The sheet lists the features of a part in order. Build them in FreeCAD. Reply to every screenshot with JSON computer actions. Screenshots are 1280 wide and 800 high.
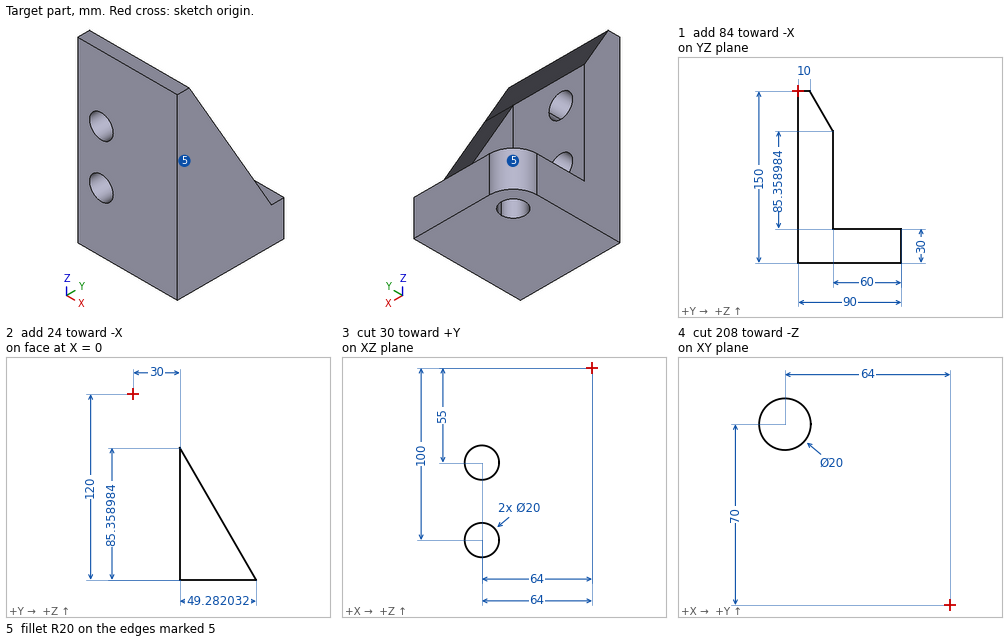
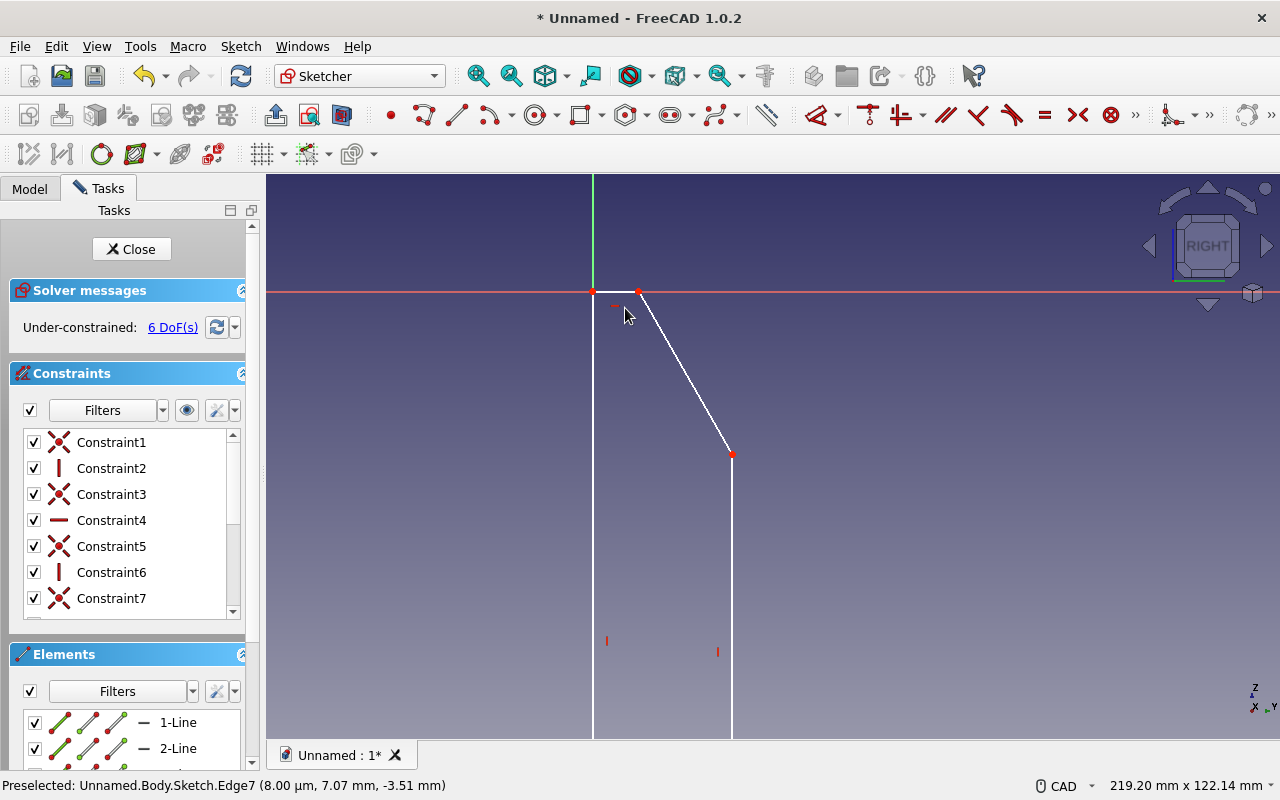
{"action": "left_click", "coordinate": [816, 116]}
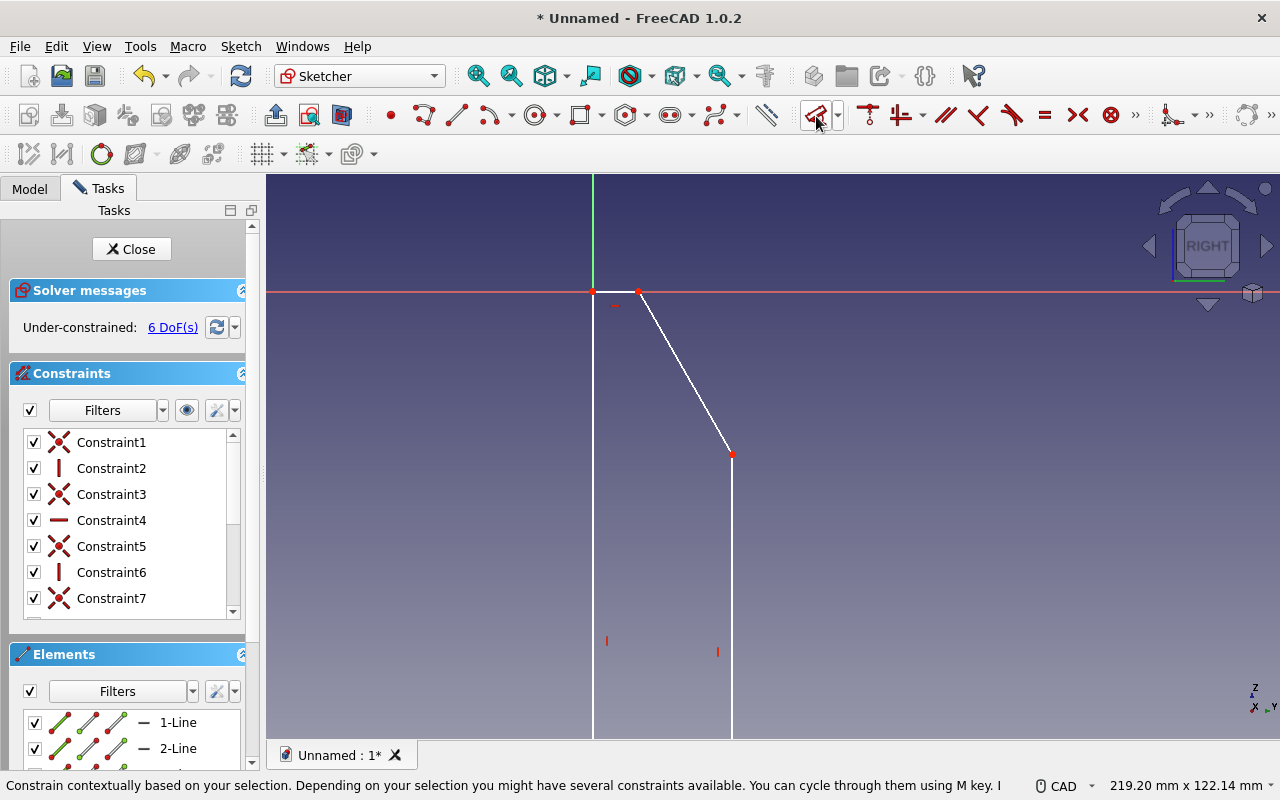
{"action": "scroll", "coordinate": [587, 235], "scroll_direction": "down", "scroll_amount": 3}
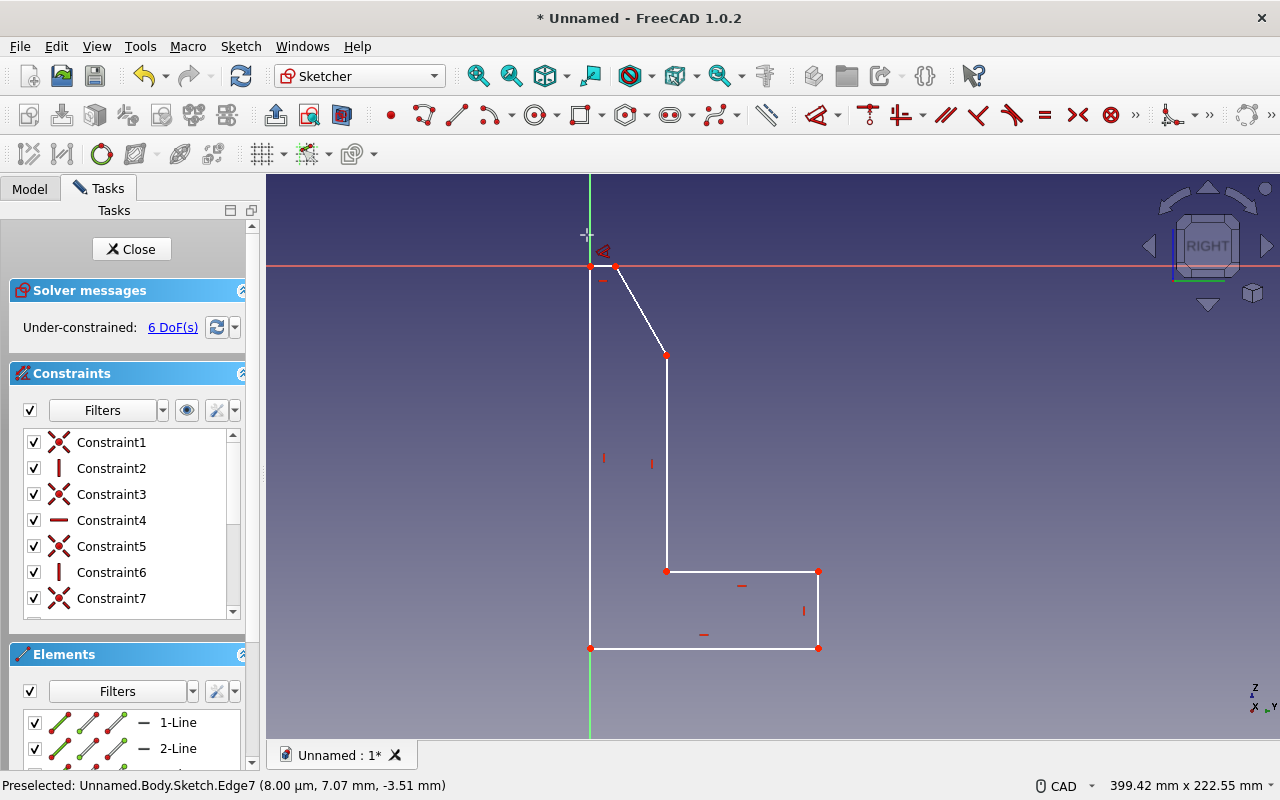
{"action": "left_click", "coordinate": [659, 649]}
{"action": "left_click", "coordinate": [704, 683]}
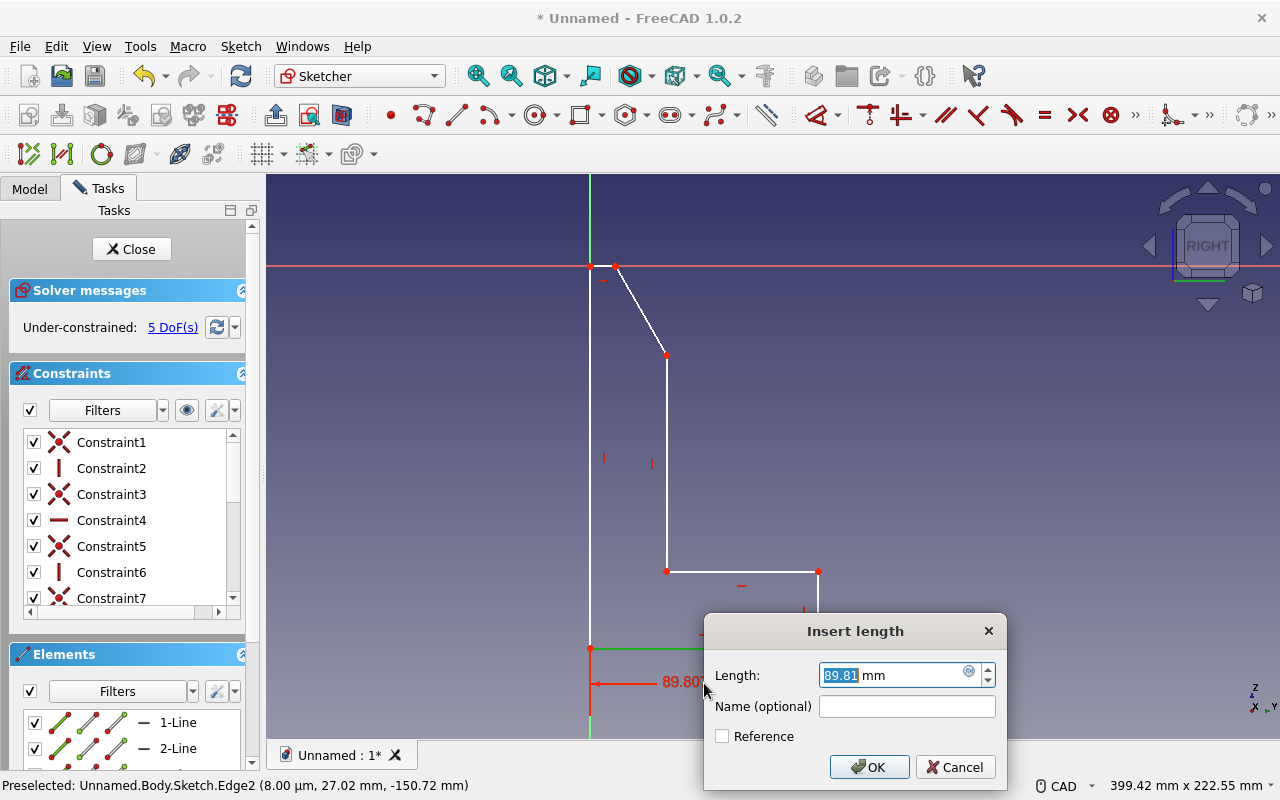
{"action": "type", "text": "90"}
{"action": "key", "text": "Return"}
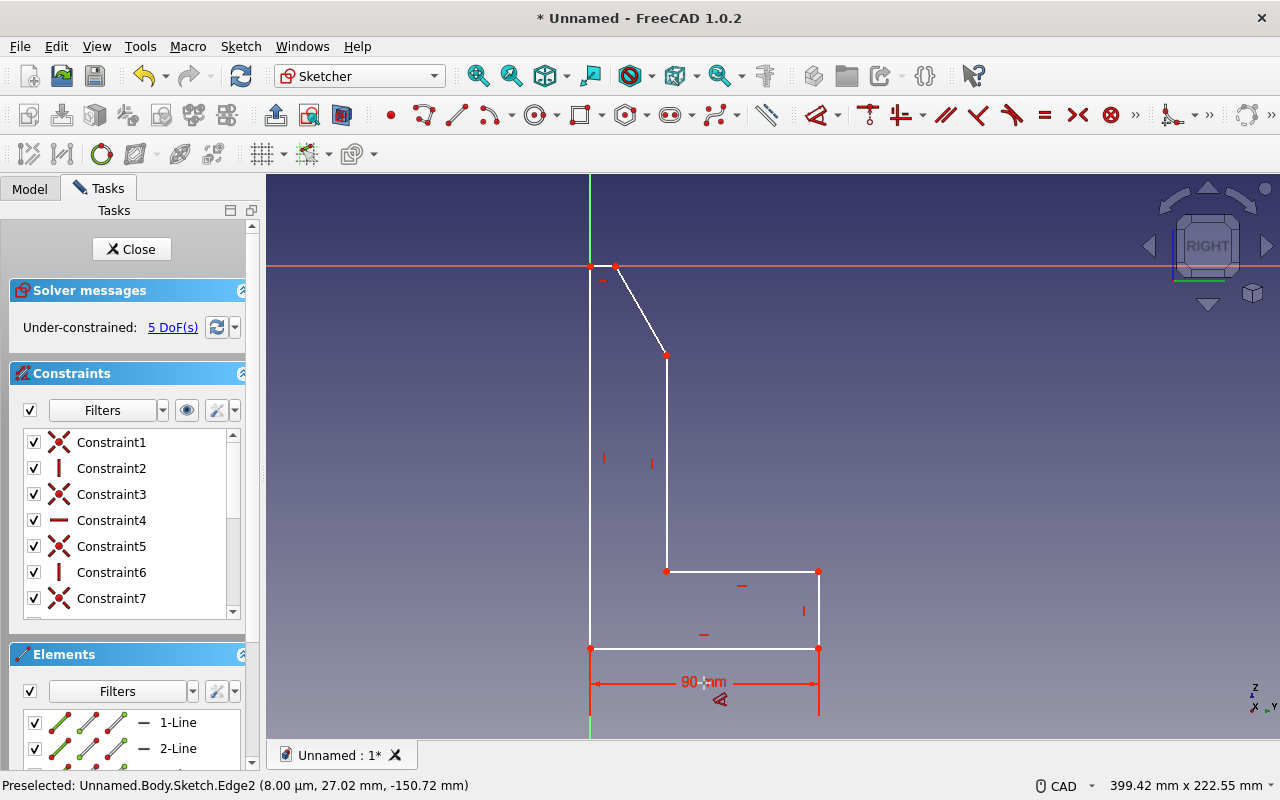
{"action": "left_click", "coordinate": [819, 626]}
{"action": "left_click", "coordinate": [853, 610]}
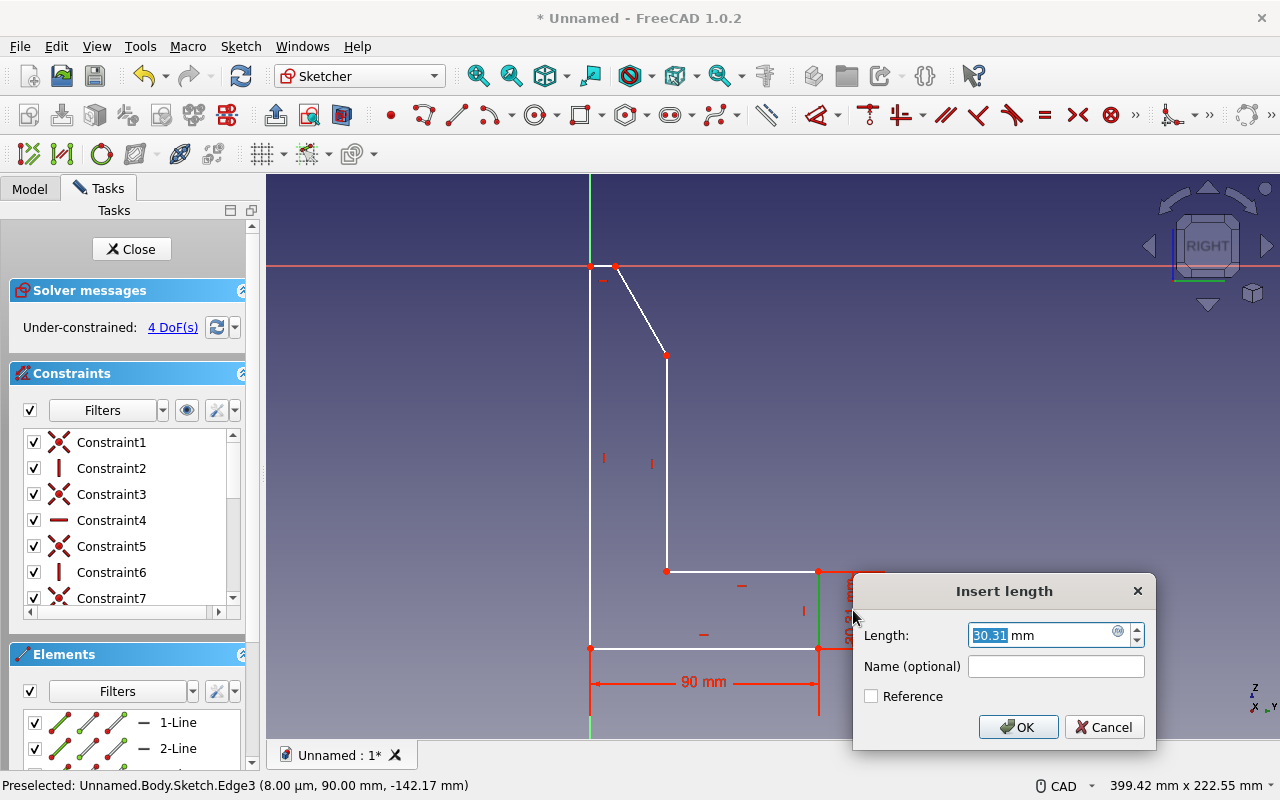
{"action": "type", "text": "30"}
{"action": "key", "text": "Return"}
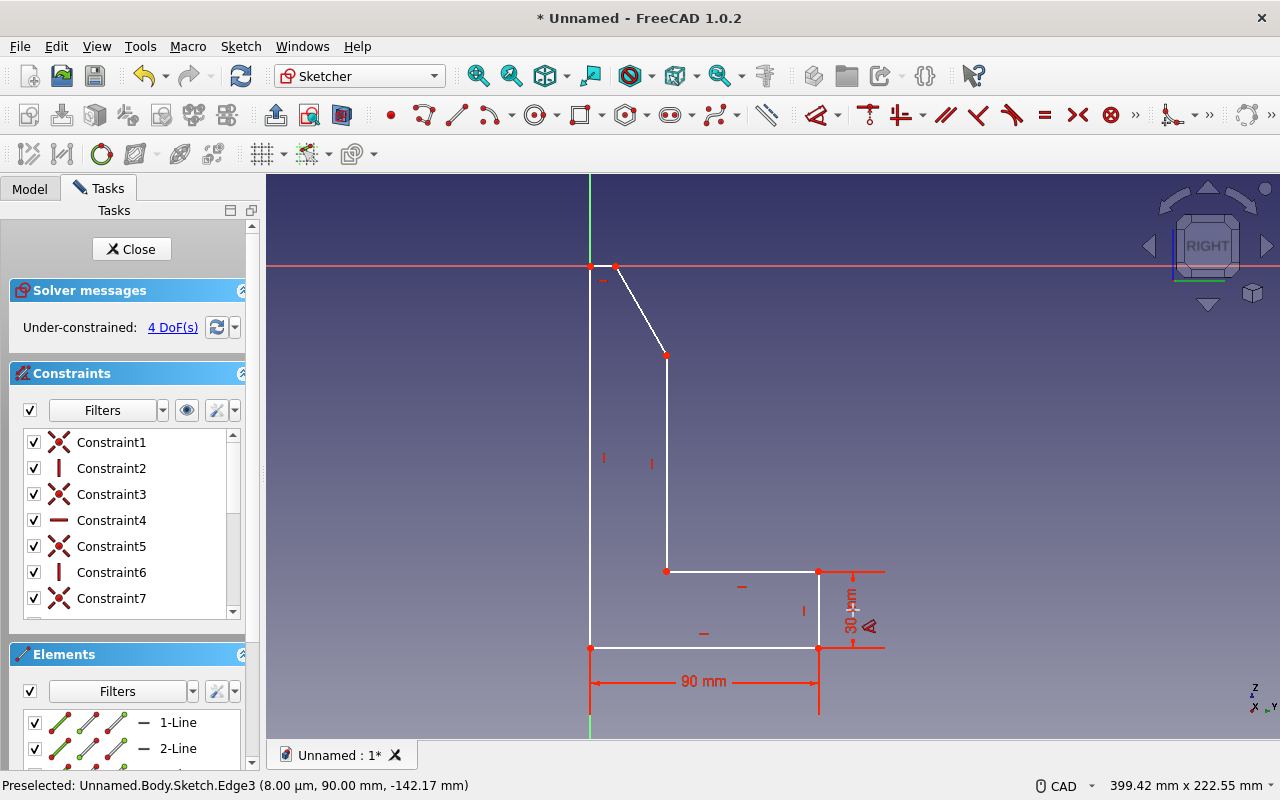
{"action": "left_click", "coordinate": [773, 572]}
{"action": "left_click", "coordinate": [743, 606]}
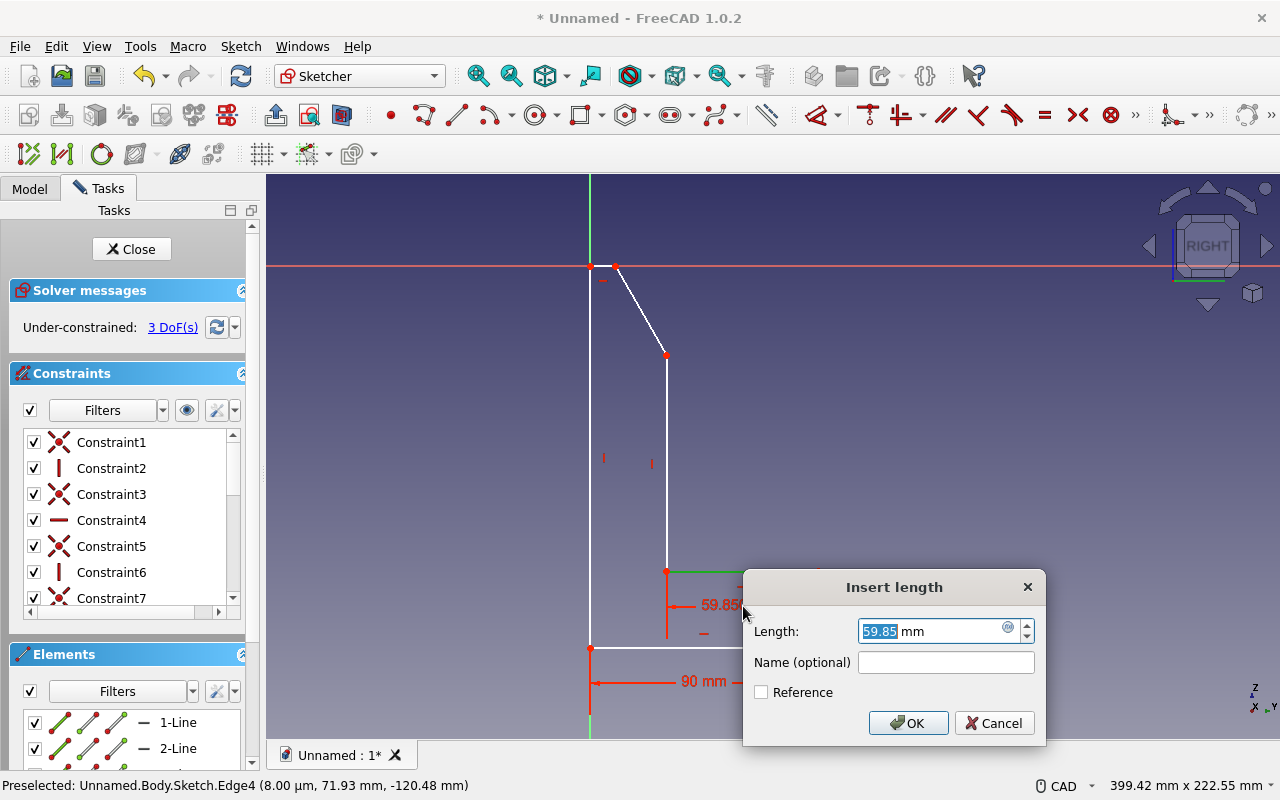
{"action": "type", "text": "60"}
{"action": "key", "text": "Return"}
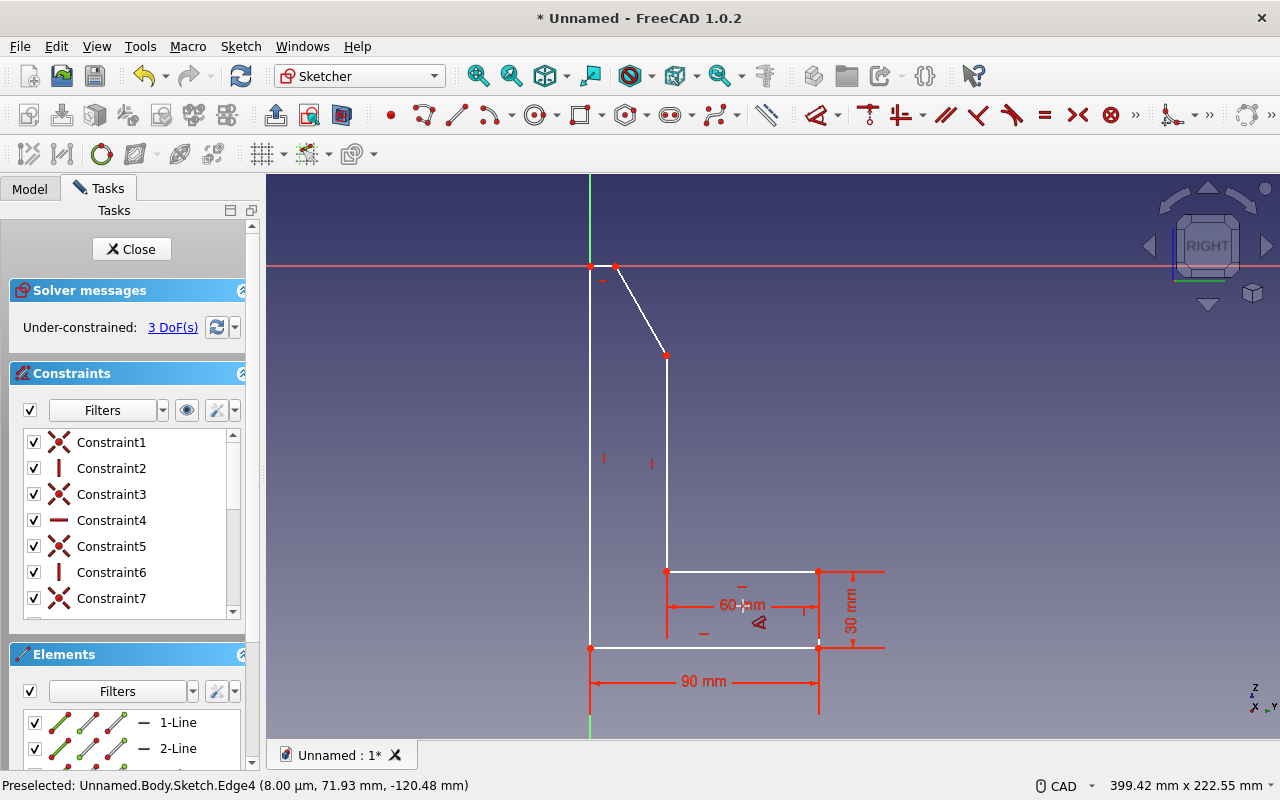
{"action": "scroll", "coordinate": [606, 266], "scroll_direction": "up", "scroll_amount": 3}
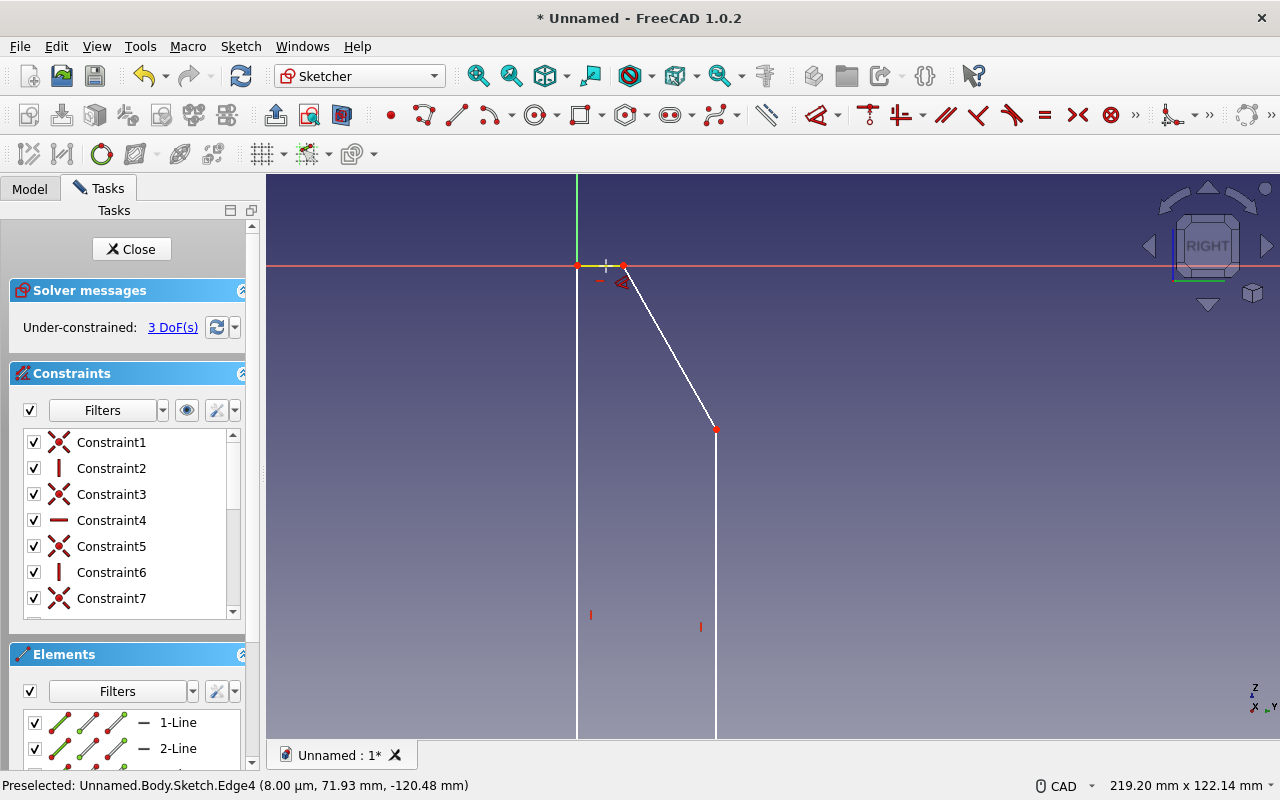
{"action": "left_click", "coordinate": [605, 266]}
{"action": "left_click", "coordinate": [600, 232]}